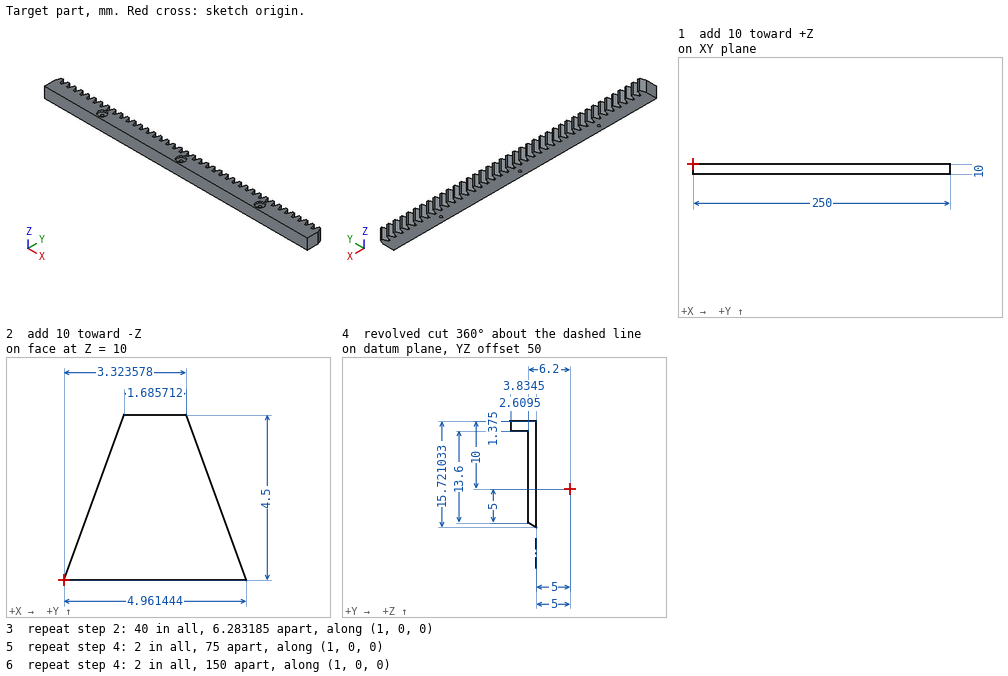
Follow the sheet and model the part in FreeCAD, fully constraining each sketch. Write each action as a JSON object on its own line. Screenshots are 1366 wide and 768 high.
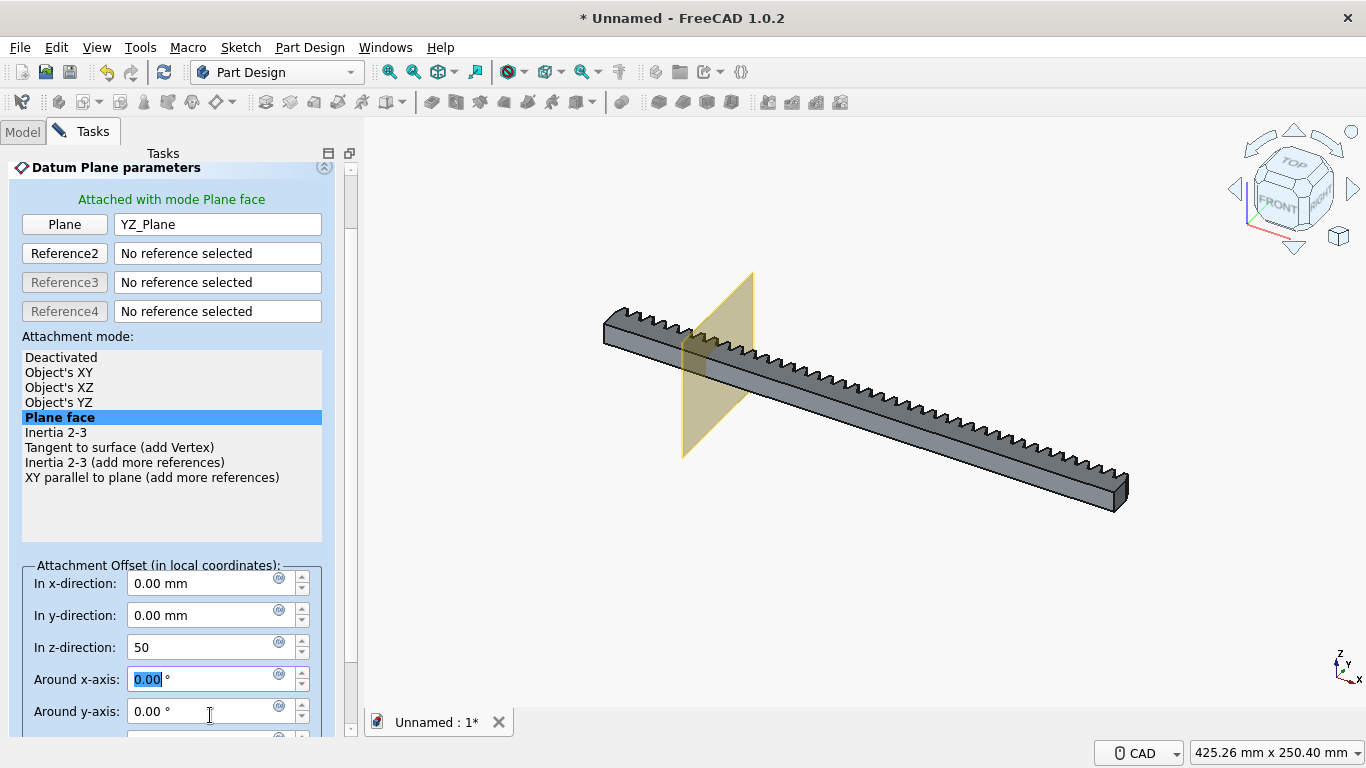
{"action": "scroll", "coordinate": [351, 450], "scroll_direction": "up", "scroll_amount": 2}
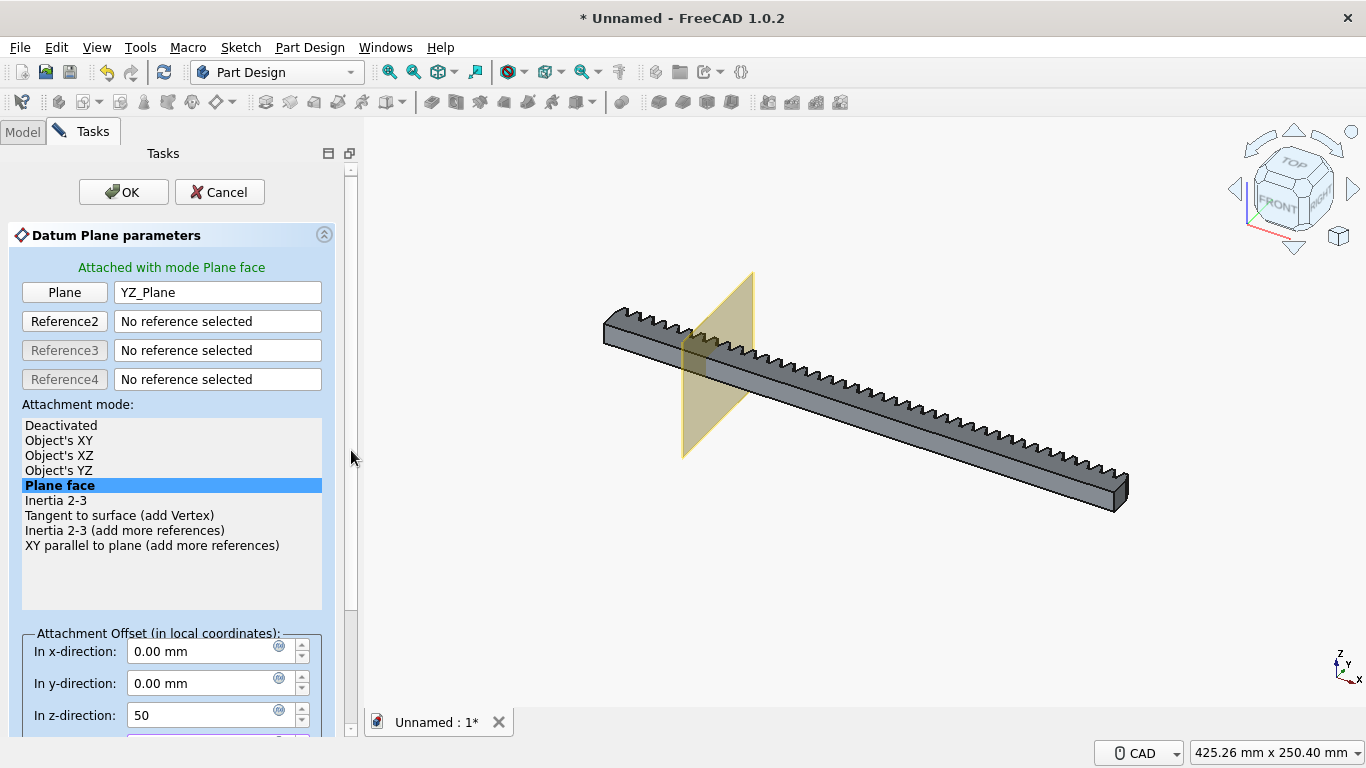
{"action": "left_click", "coordinate": [124, 192]}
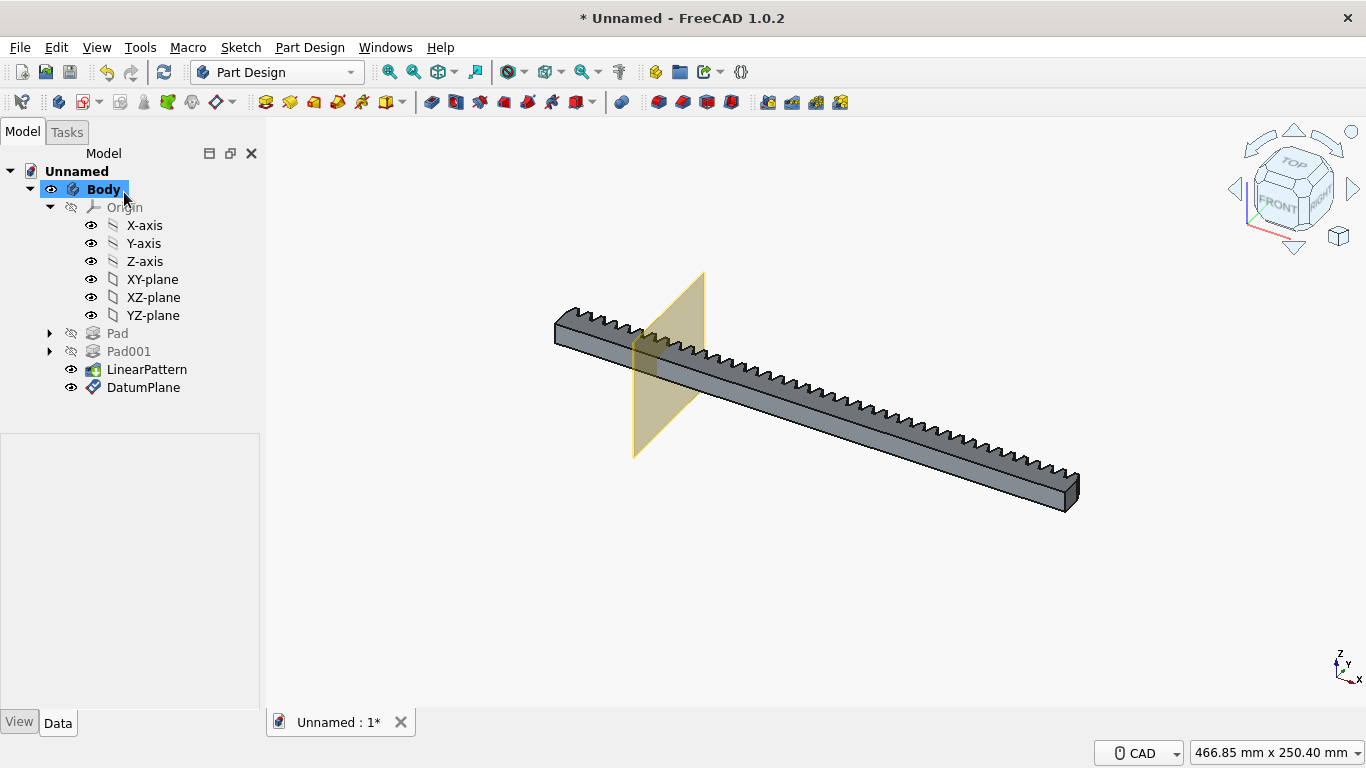
{"action": "left_click", "coordinate": [116, 387]}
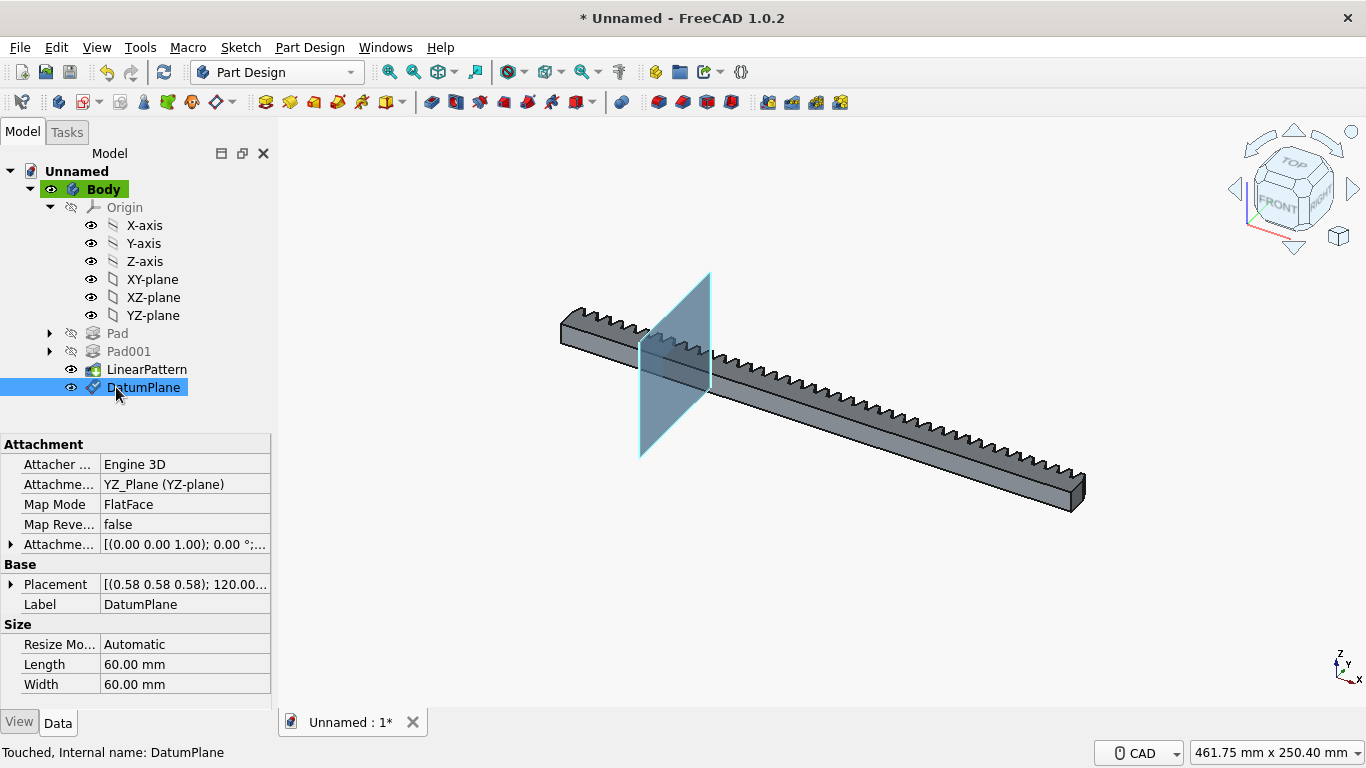
{"action": "left_click", "coordinate": [84, 102]}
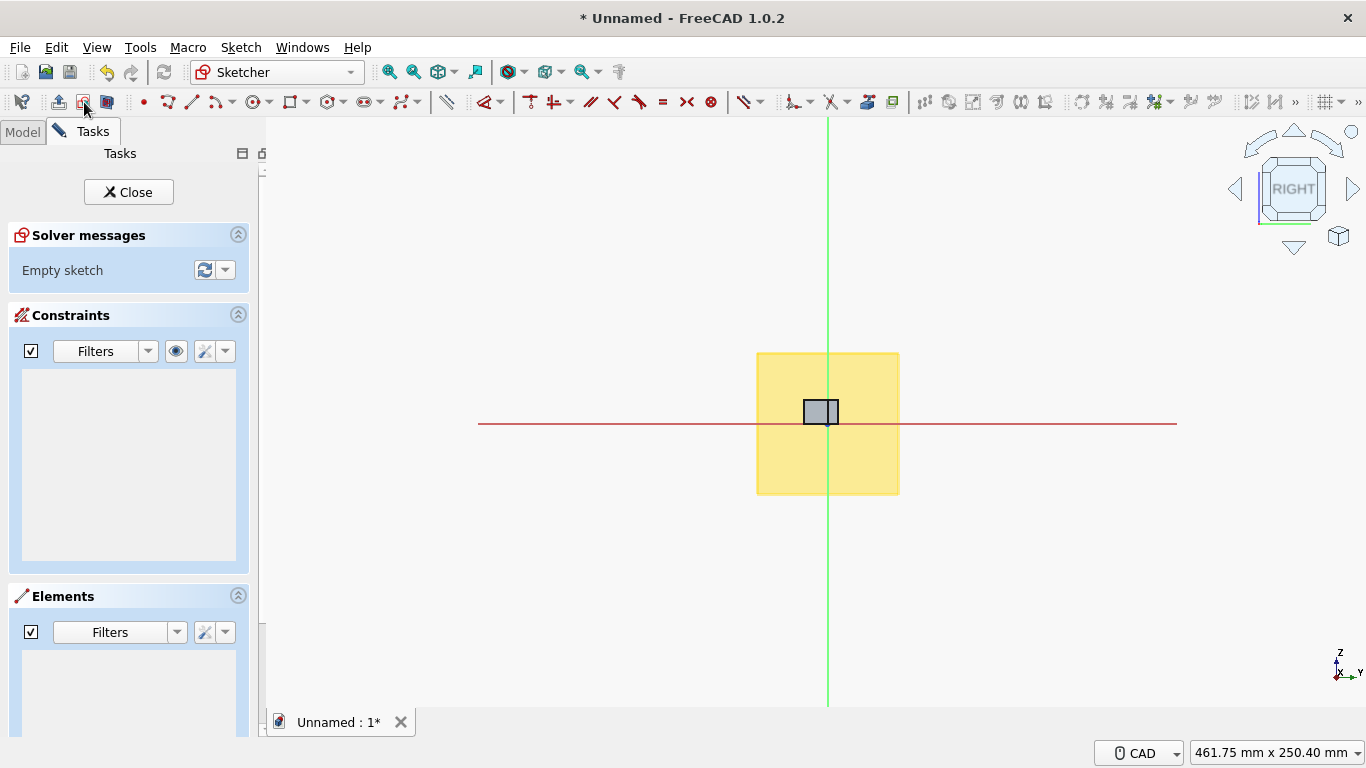
{"action": "key", "text": "q s"}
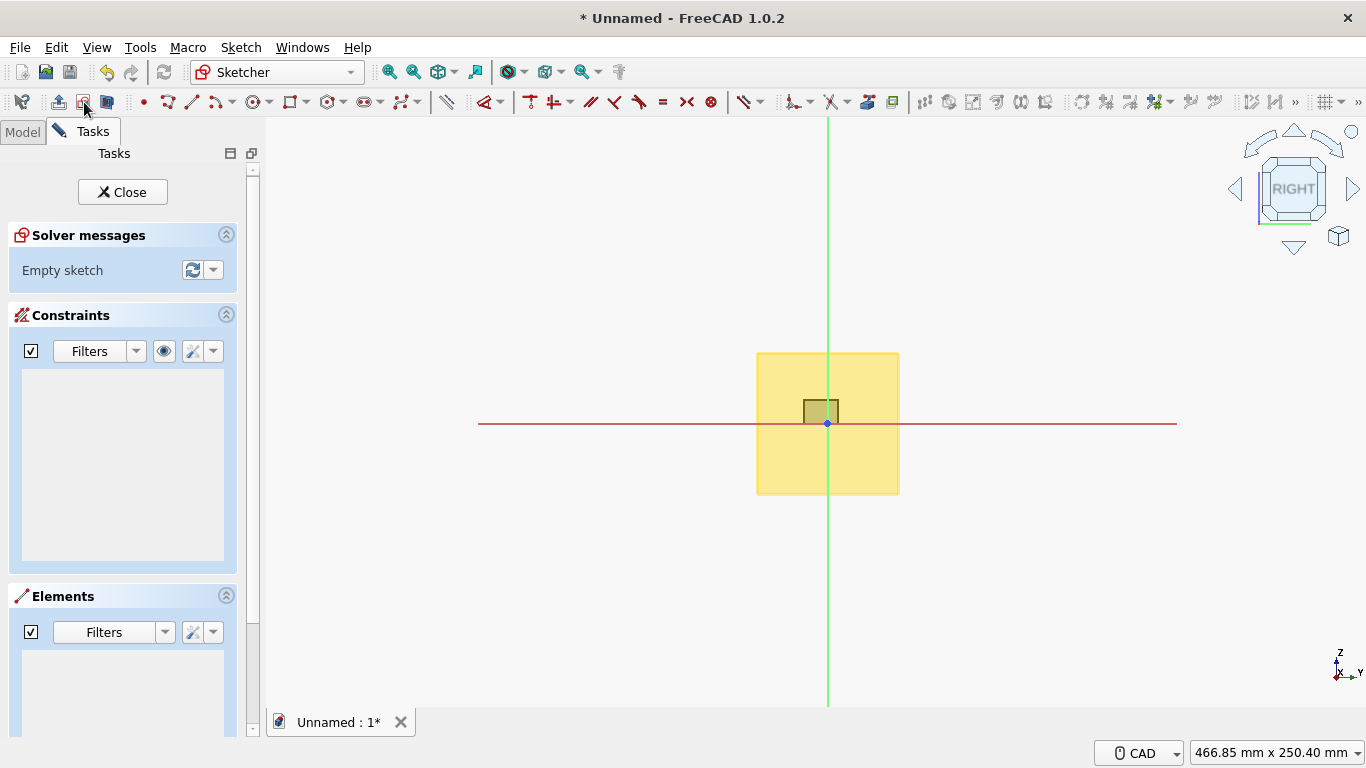
{"action": "scroll", "coordinate": [828, 428], "scroll_direction": "up", "scroll_amount": 10}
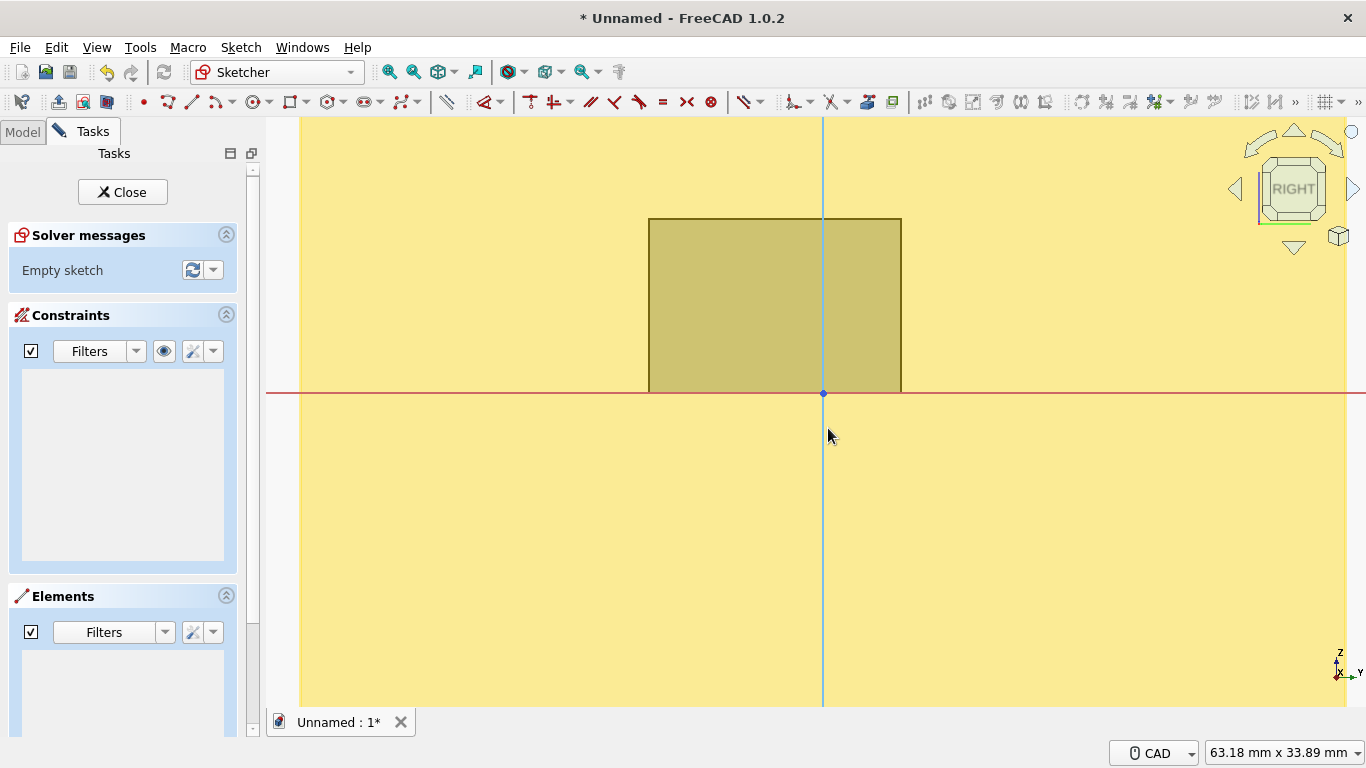
{"action": "key", "text": "g m"}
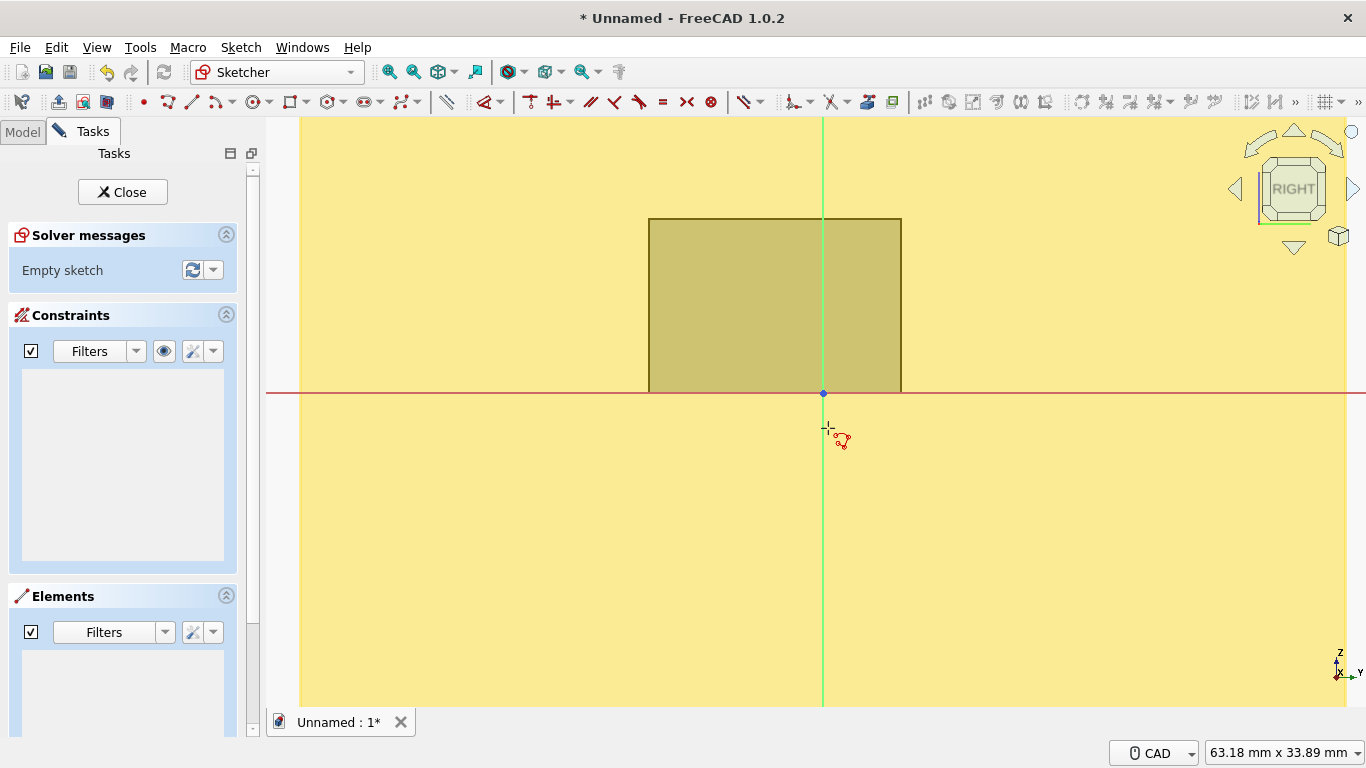
{"action": "left_click", "coordinate": [736, 493]}
{"action": "left_click", "coordinate": [736, 219]}
{"action": "left_click", "coordinate": [669, 219]}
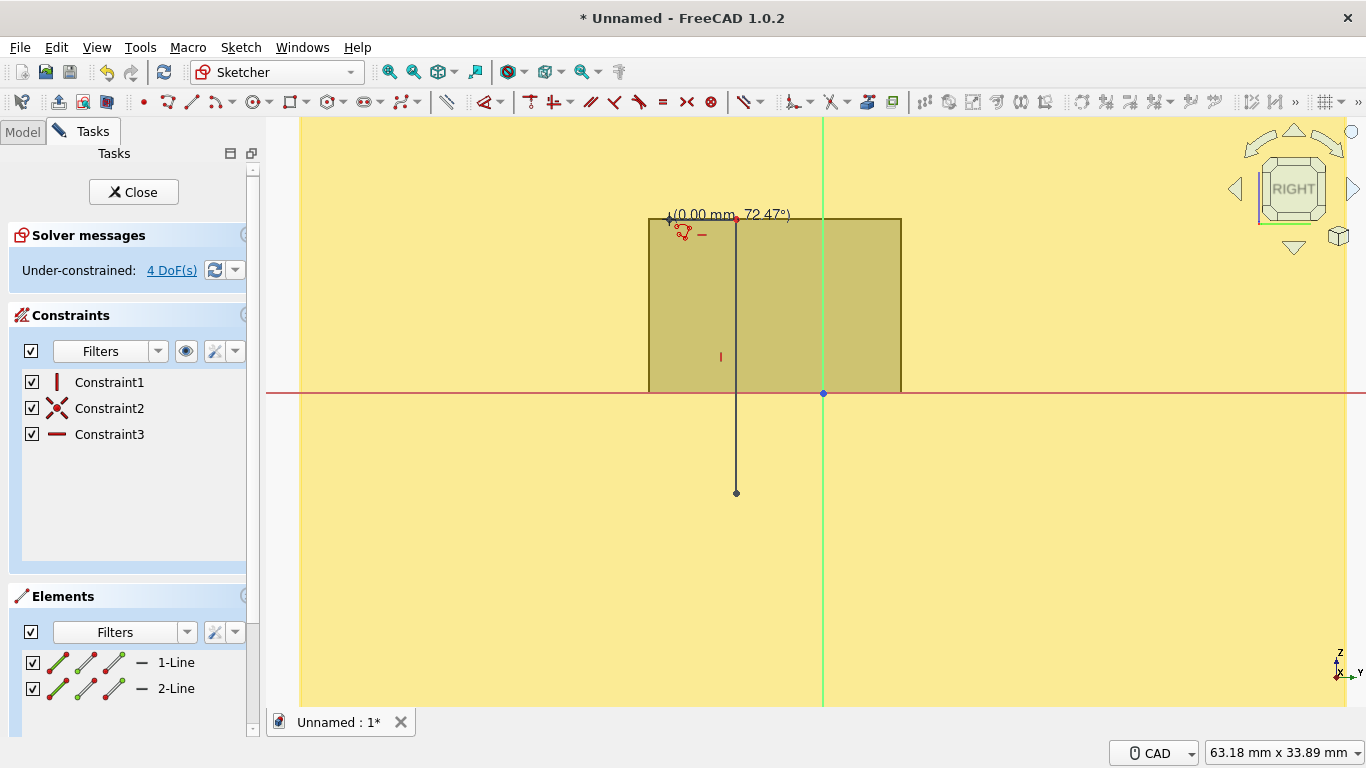
{"action": "scroll", "coordinate": [670, 220], "scroll_direction": "up", "scroll_amount": 18}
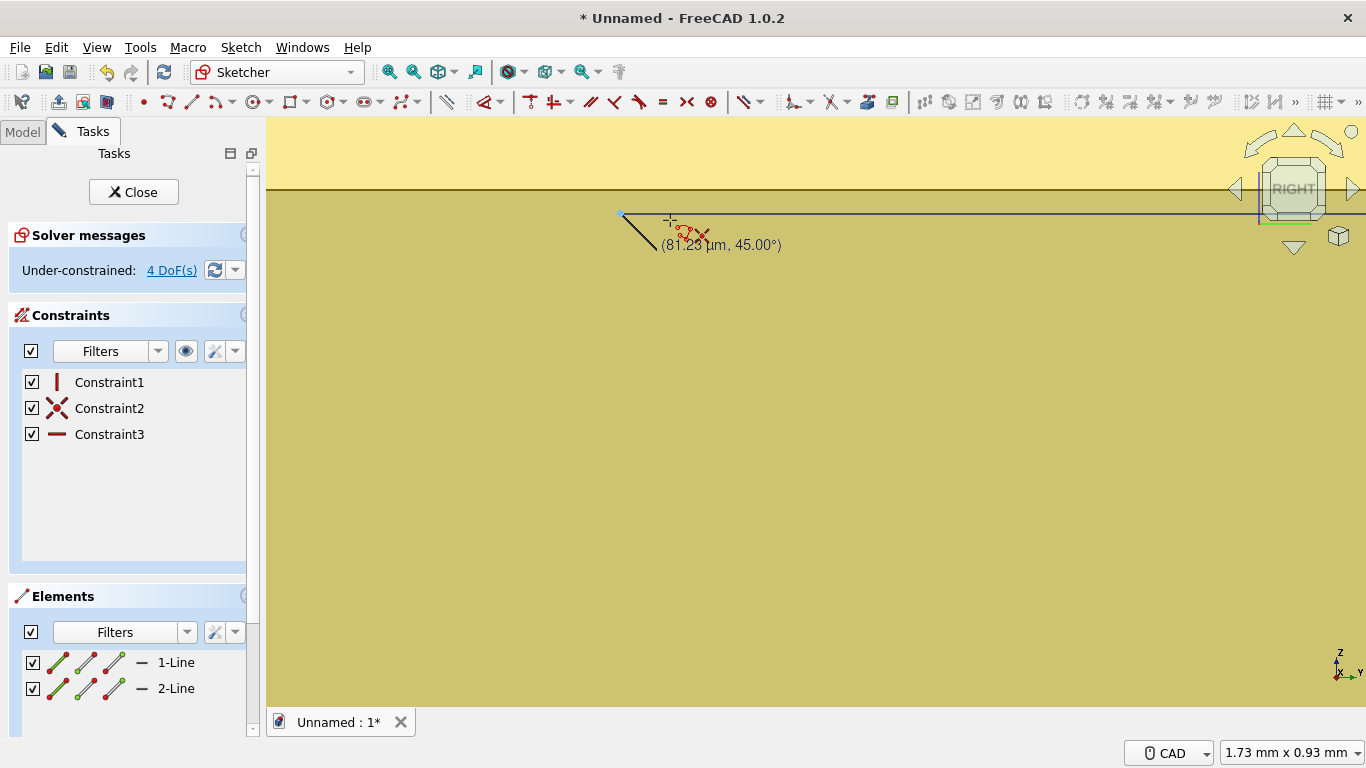
{"action": "left_click", "coordinate": [647, 206]}